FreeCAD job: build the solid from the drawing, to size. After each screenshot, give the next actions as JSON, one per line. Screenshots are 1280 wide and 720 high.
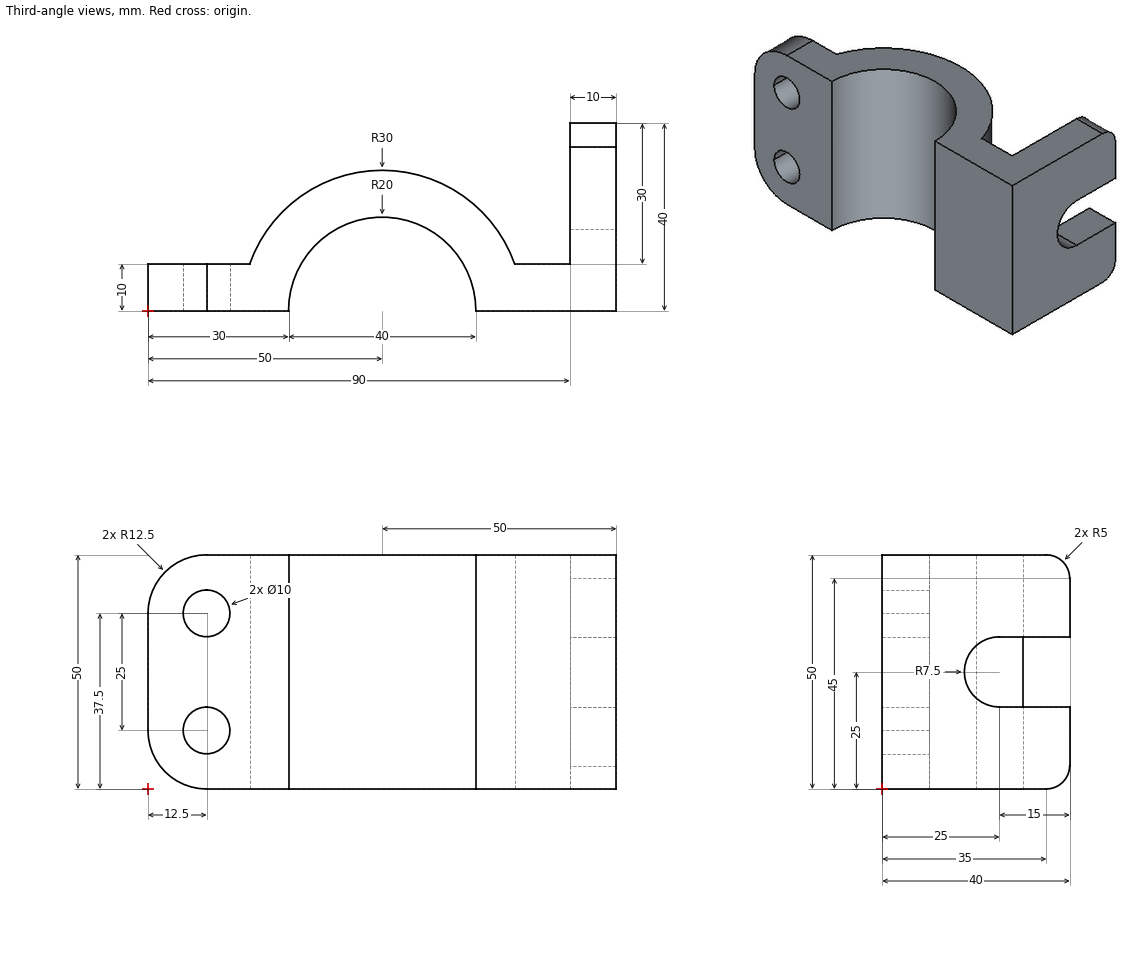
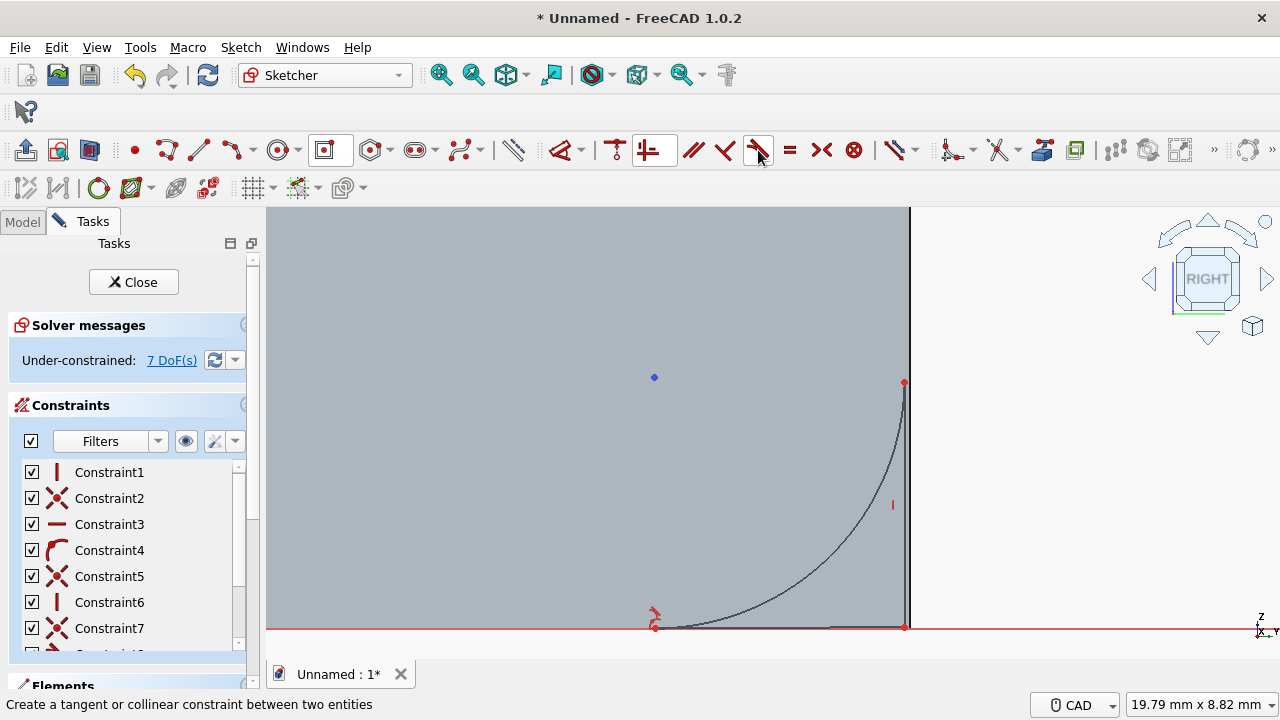
{"action": "scroll", "coordinate": [807, 568], "scroll_direction": "down", "scroll_amount": 11}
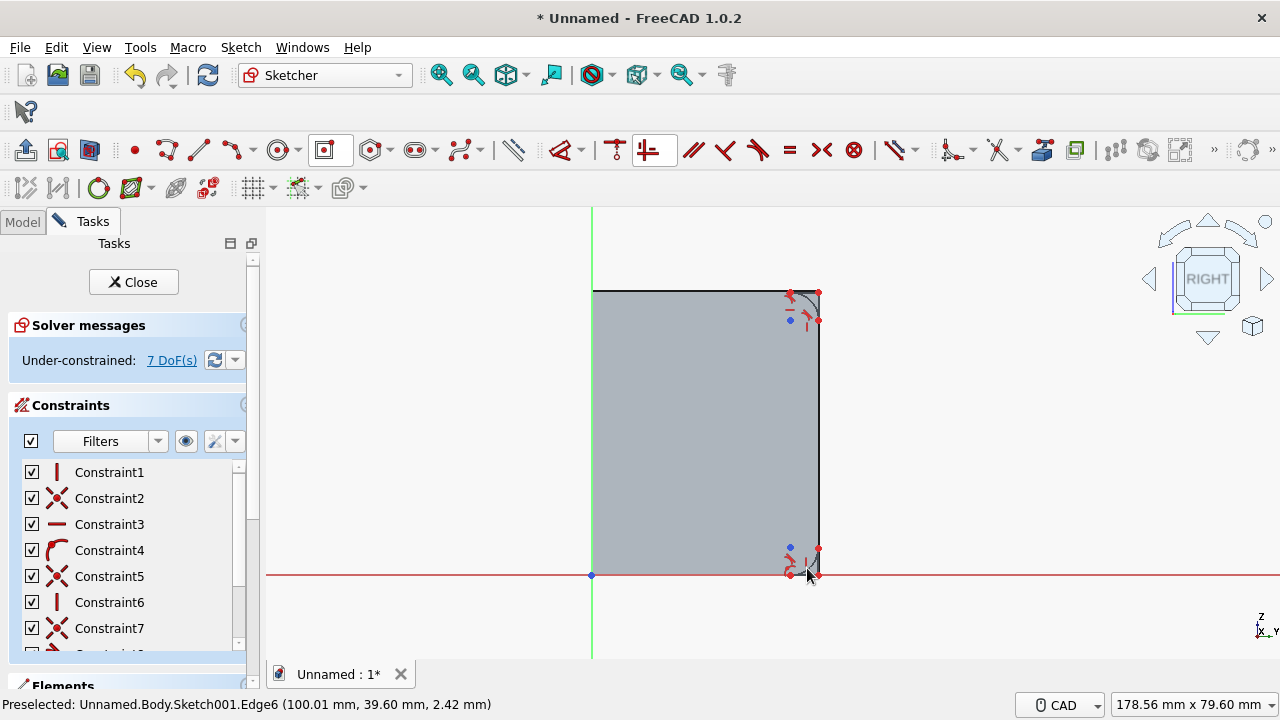
{"action": "scroll", "coordinate": [818, 567], "scroll_direction": "up", "scroll_amount": 5}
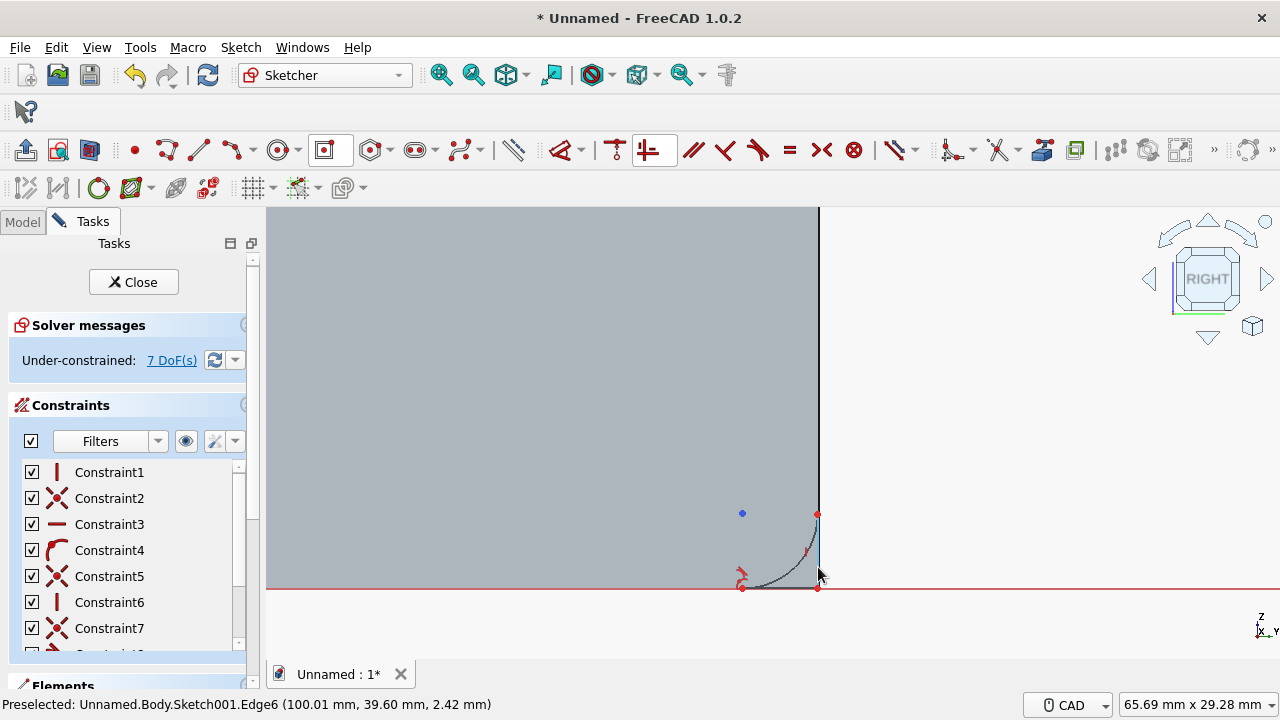
{"action": "left_click", "coordinate": [818, 566]}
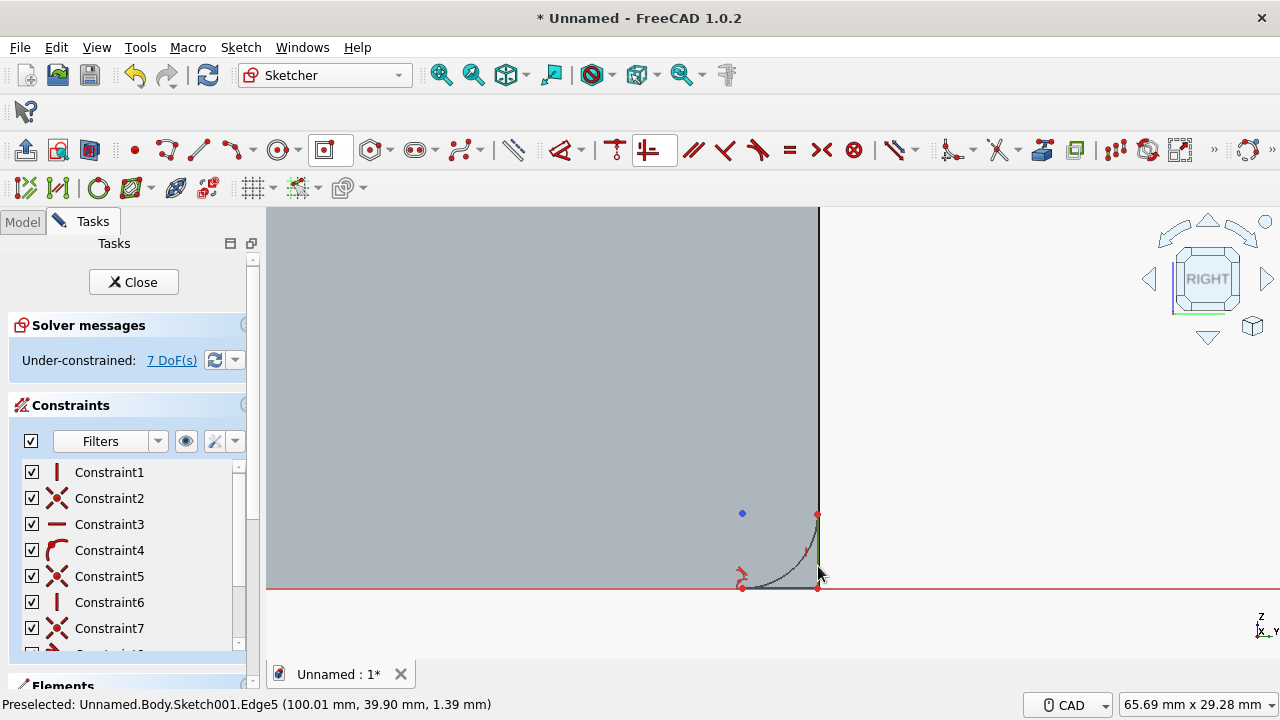
{"action": "left_click", "coordinate": [795, 567]}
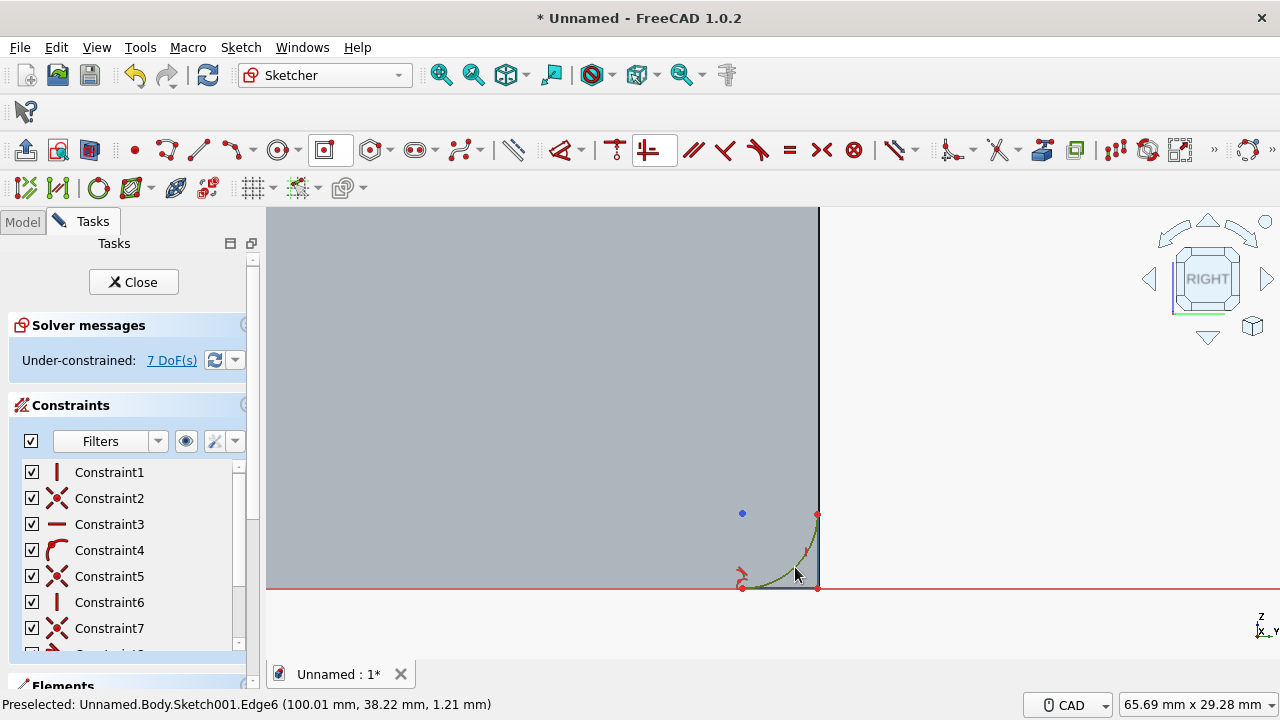
{"action": "left_click", "coordinate": [758, 150]}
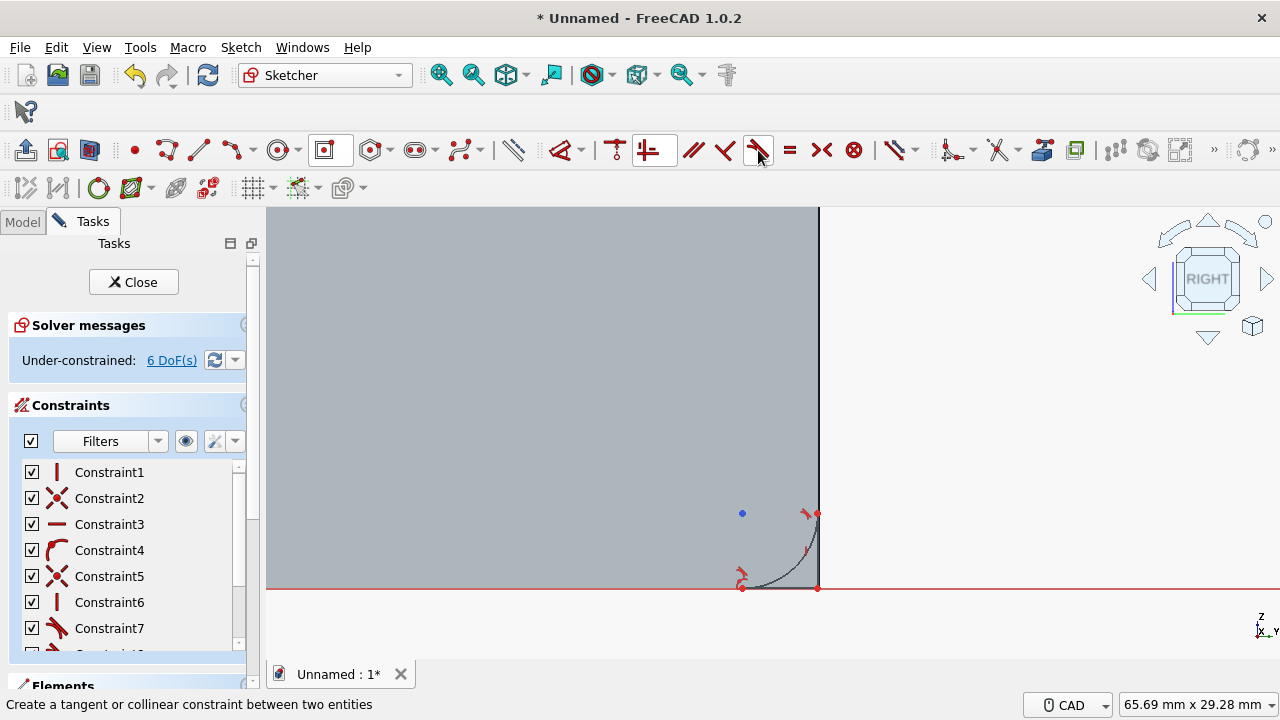
{"action": "left_click", "coordinate": [795, 588]}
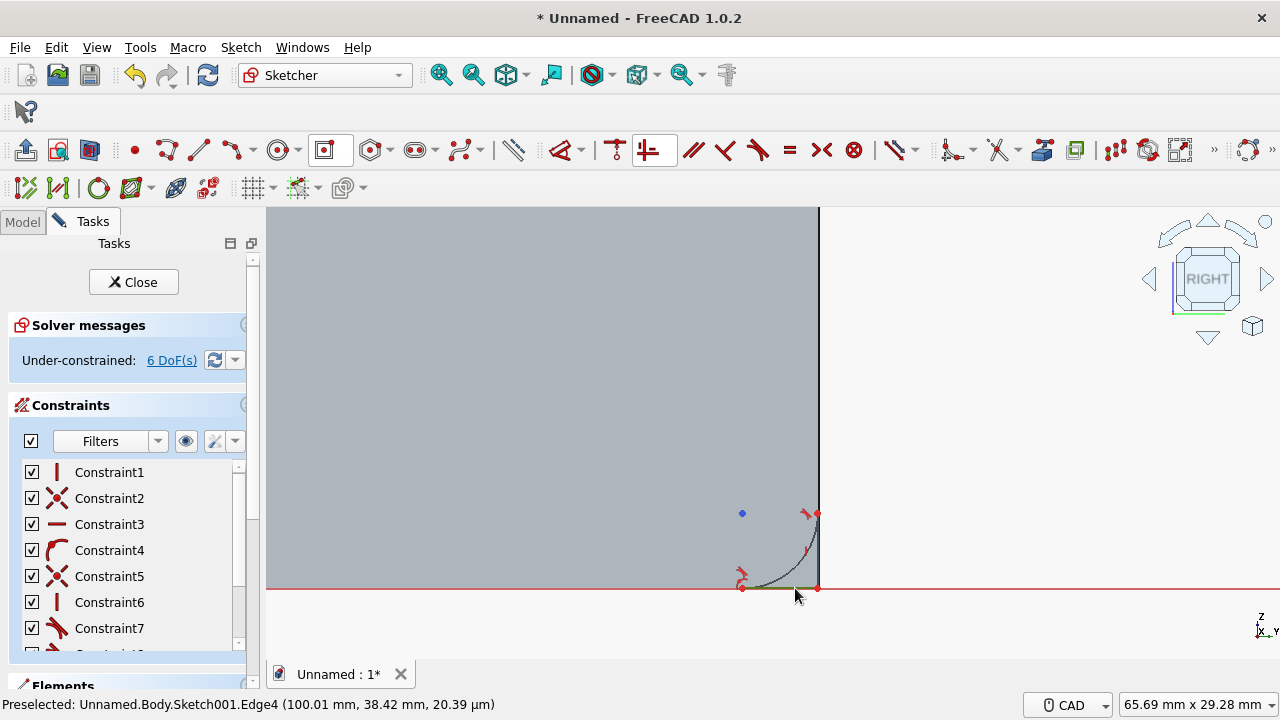
{"action": "left_click", "coordinate": [672, 150]}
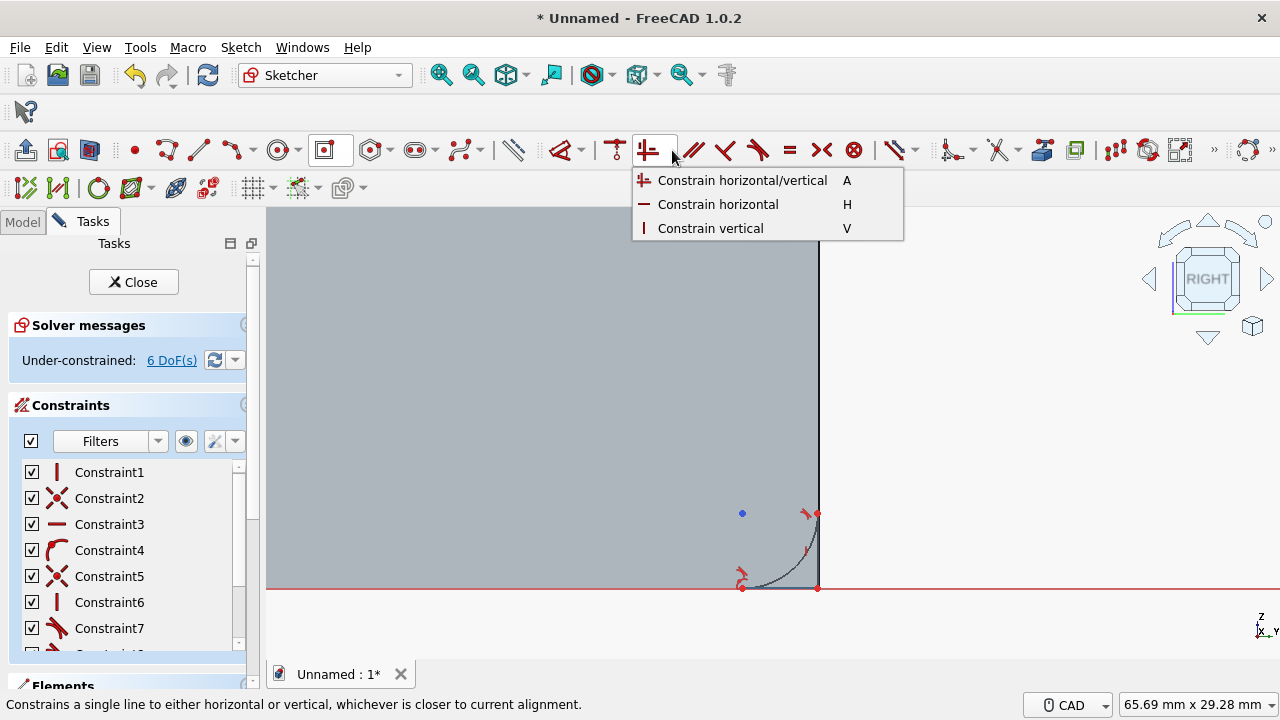
{"action": "left_click", "coordinate": [768, 204]}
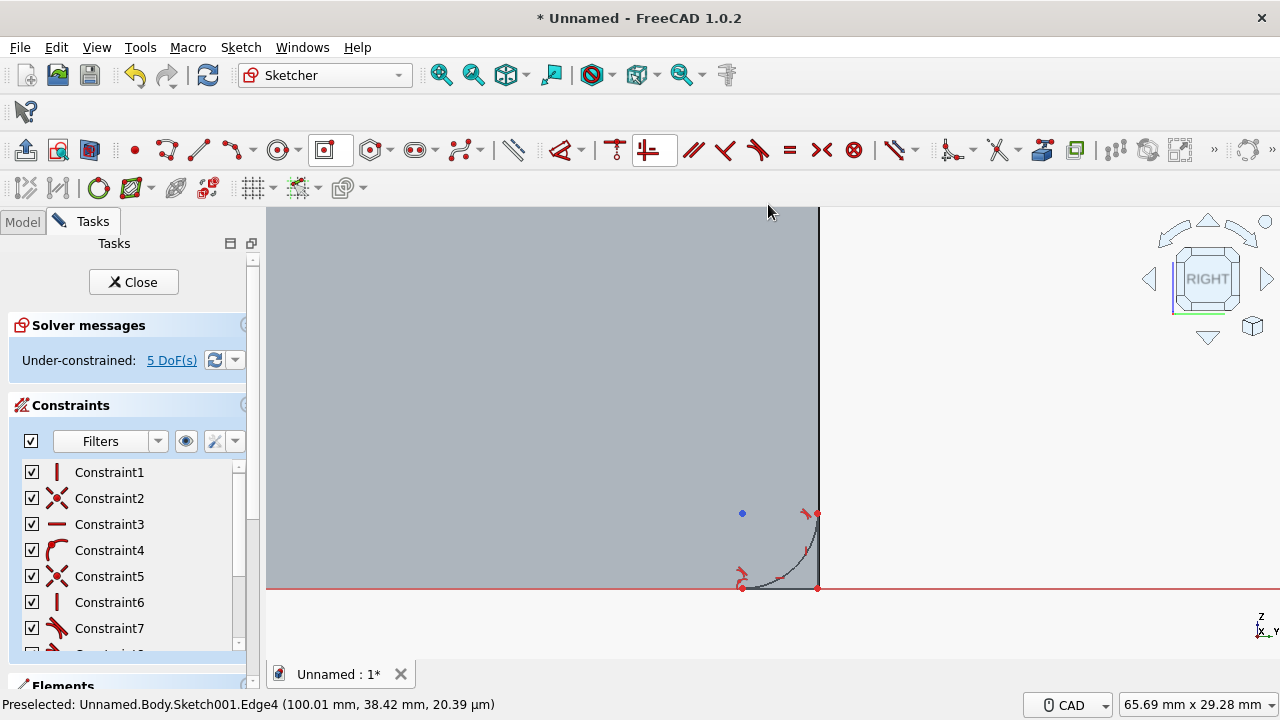
{"action": "scroll", "coordinate": [817, 567], "scroll_direction": "down", "scroll_amount": 5}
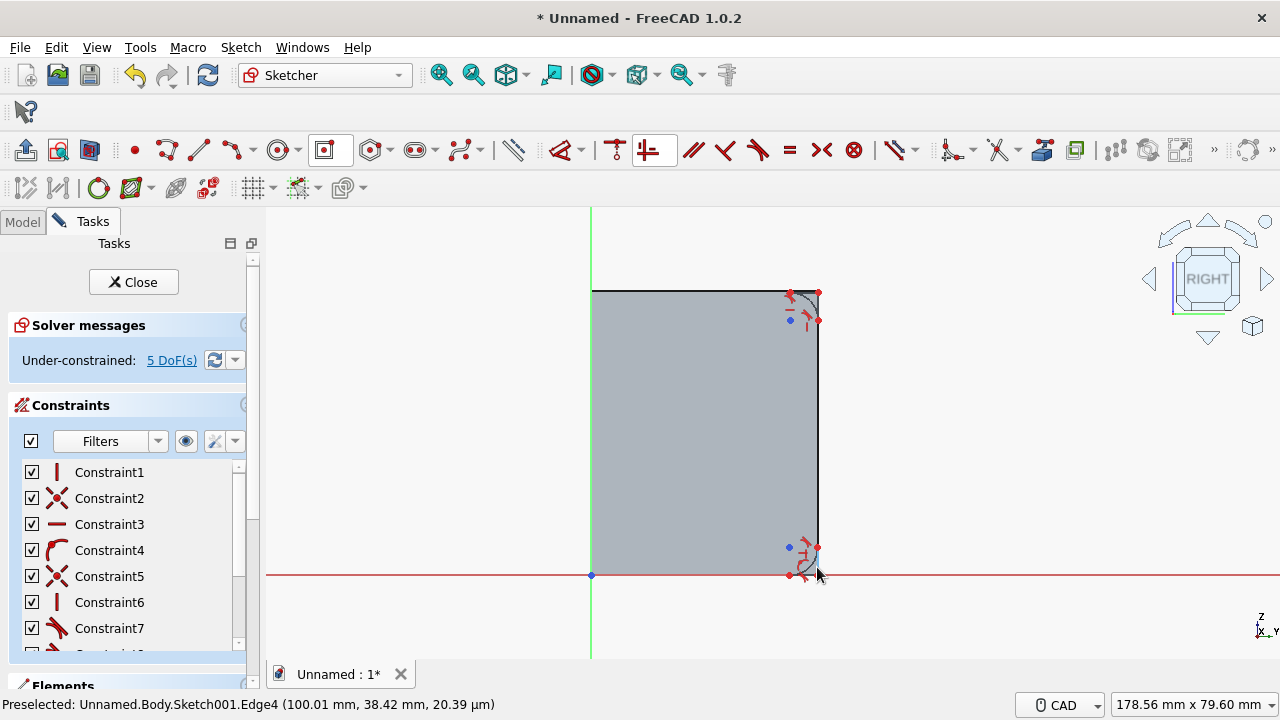
{"action": "scroll", "coordinate": [810, 301], "scroll_direction": "up", "scroll_amount": 3}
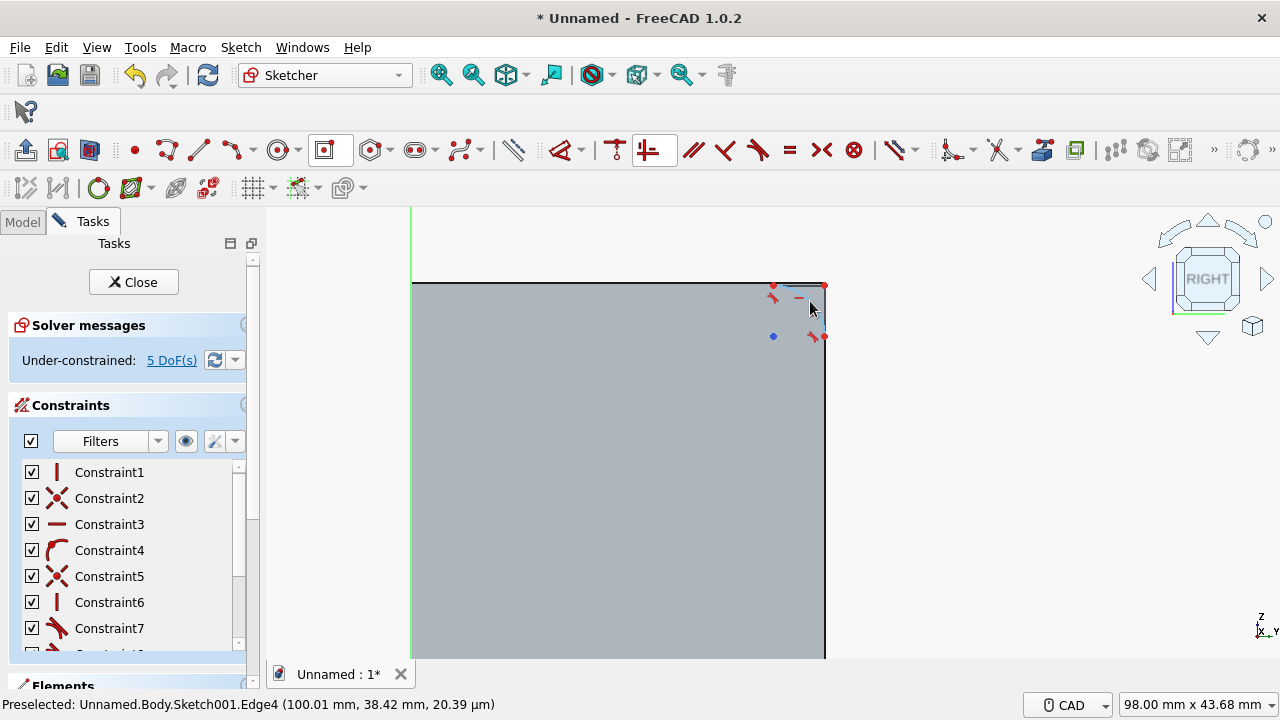
{"action": "left_click", "coordinate": [810, 301]}